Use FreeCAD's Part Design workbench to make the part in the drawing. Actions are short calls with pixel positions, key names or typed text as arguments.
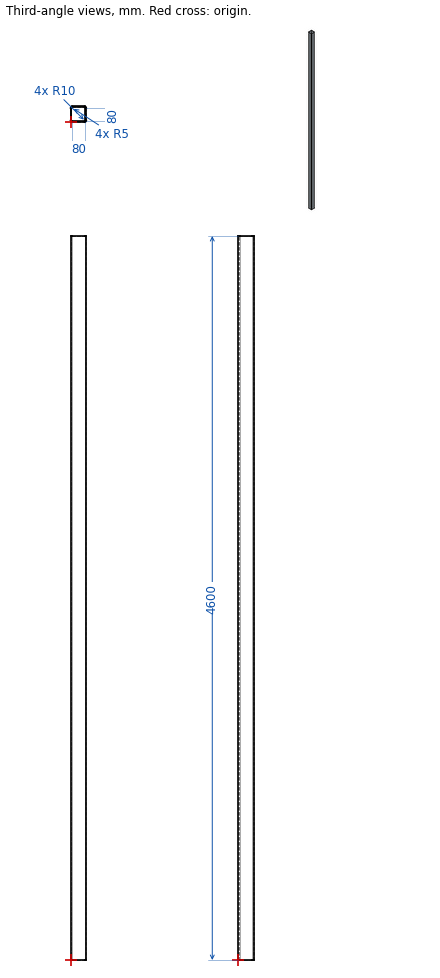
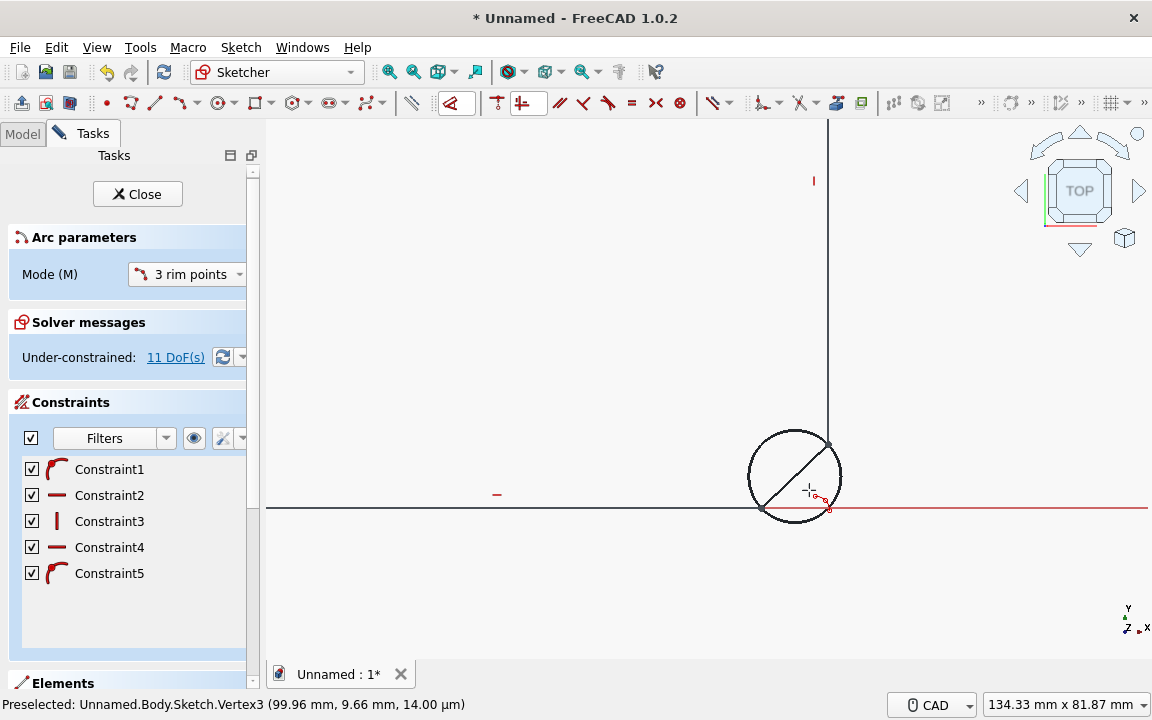
click(809, 489)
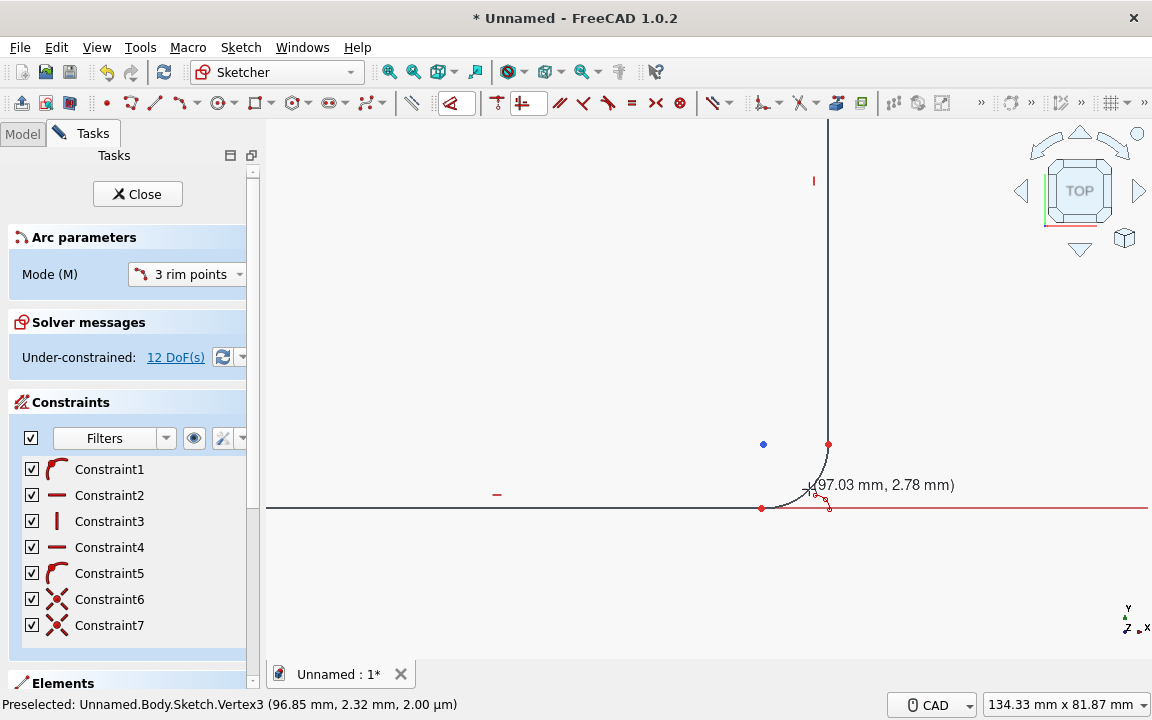
scroll(813, 631, down, 3)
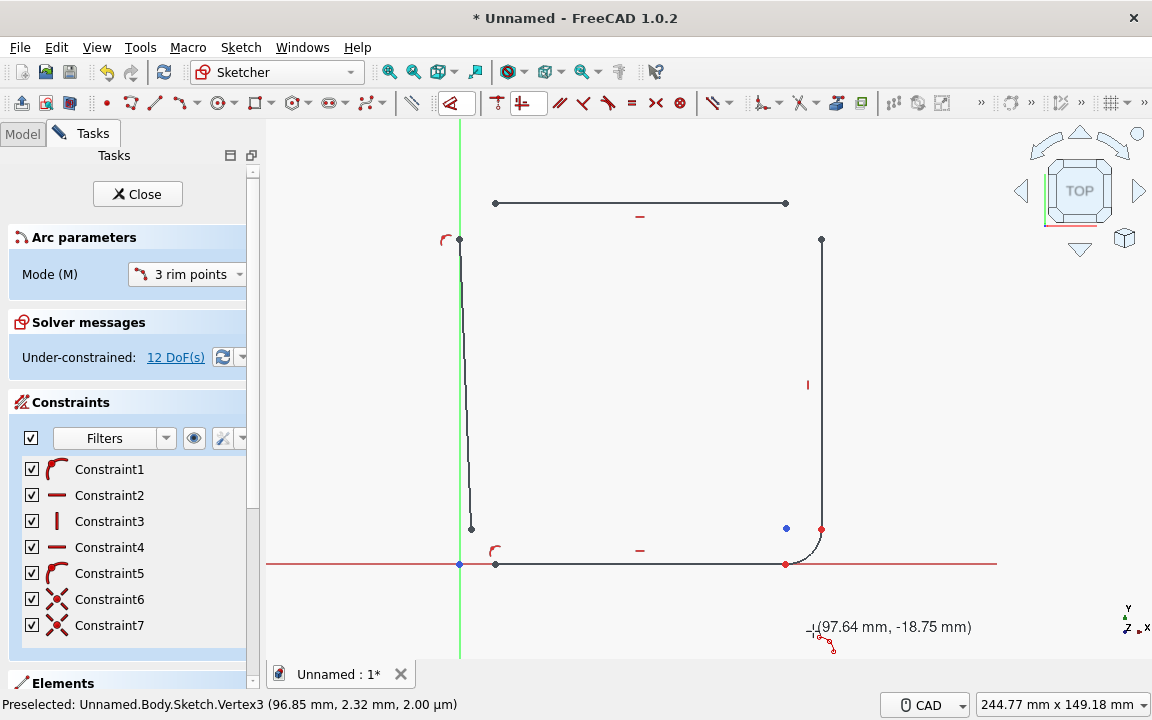
click(822, 240)
click(785, 203)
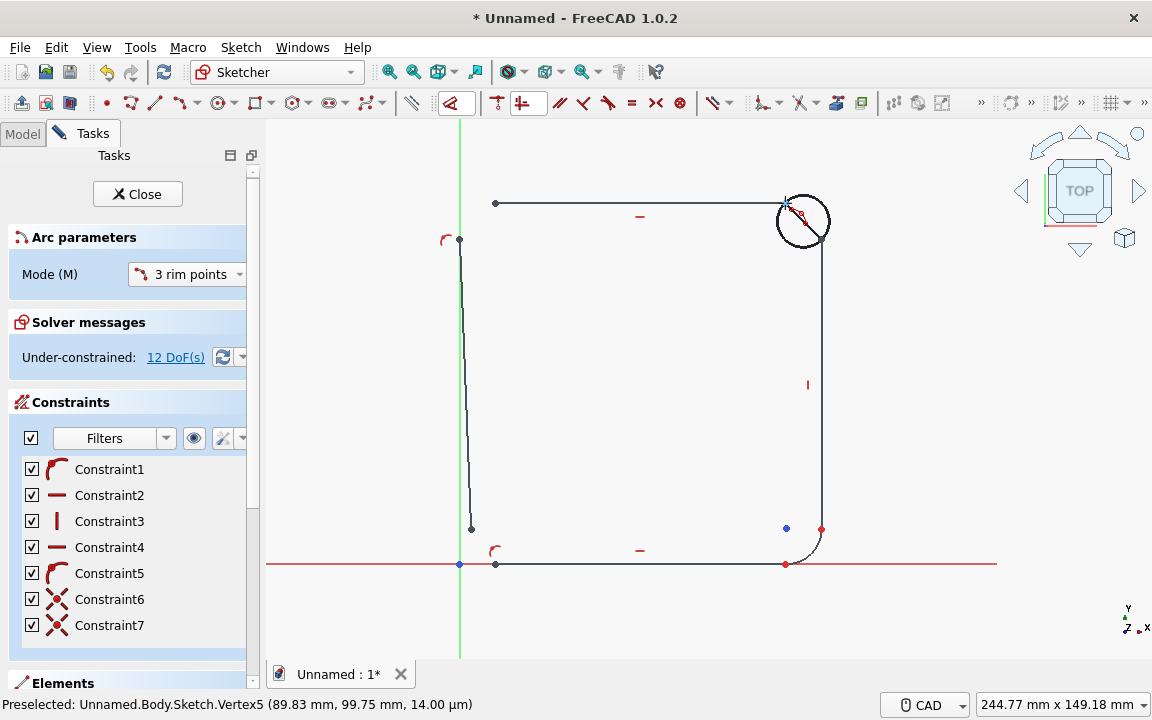
scroll(811, 213, up, 3)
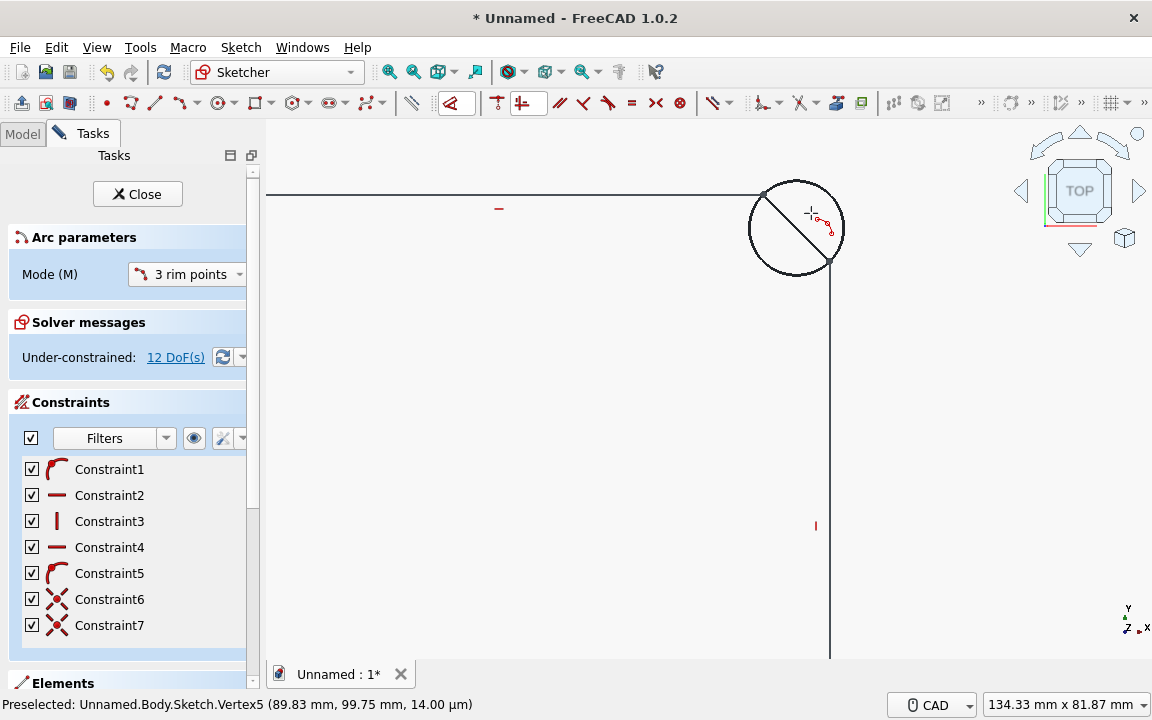
click(811, 212)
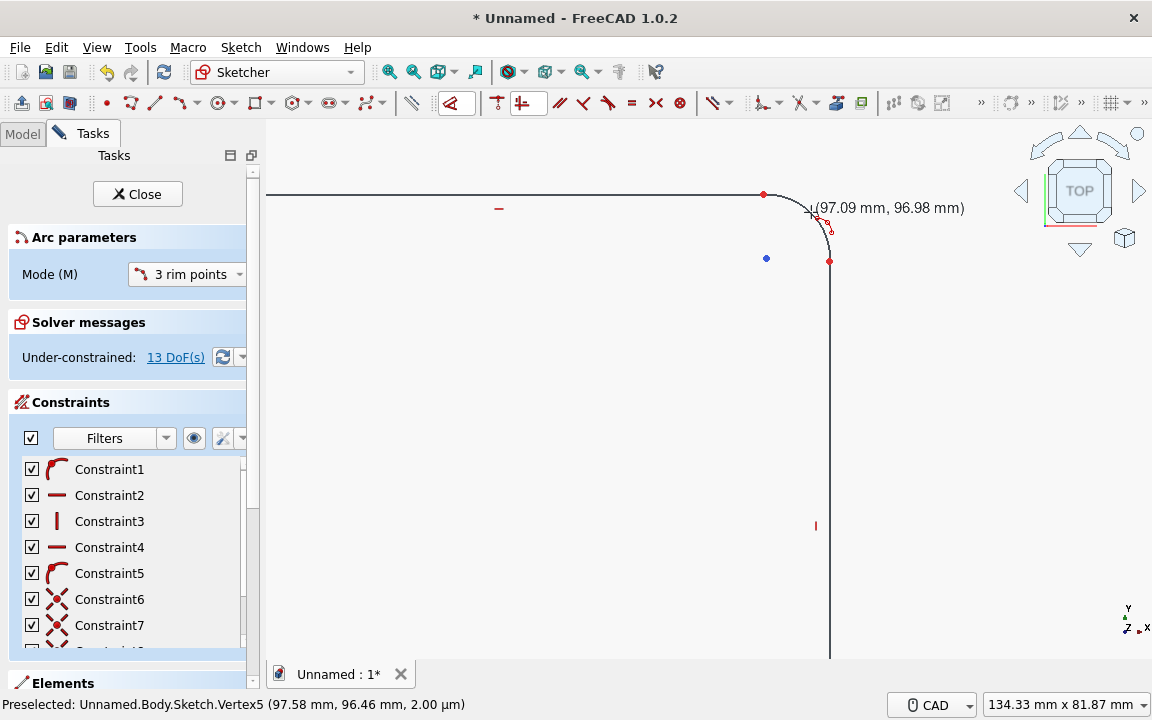
scroll(811, 226, down, 3)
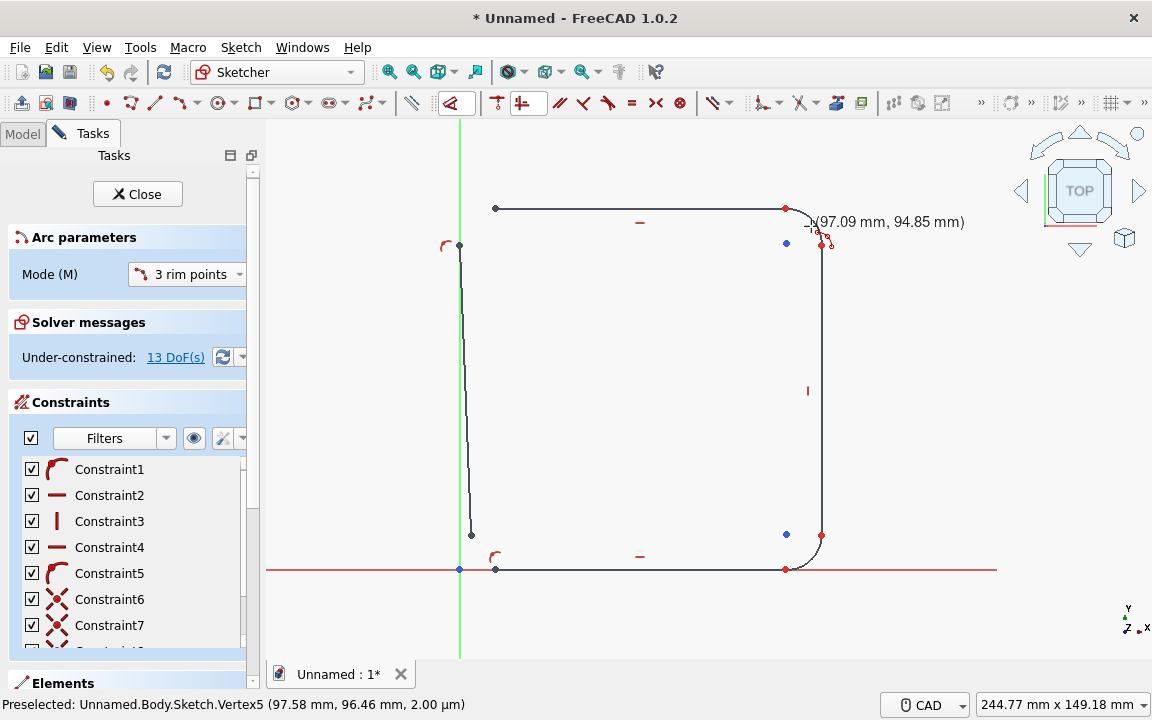
click(496, 209)
click(460, 246)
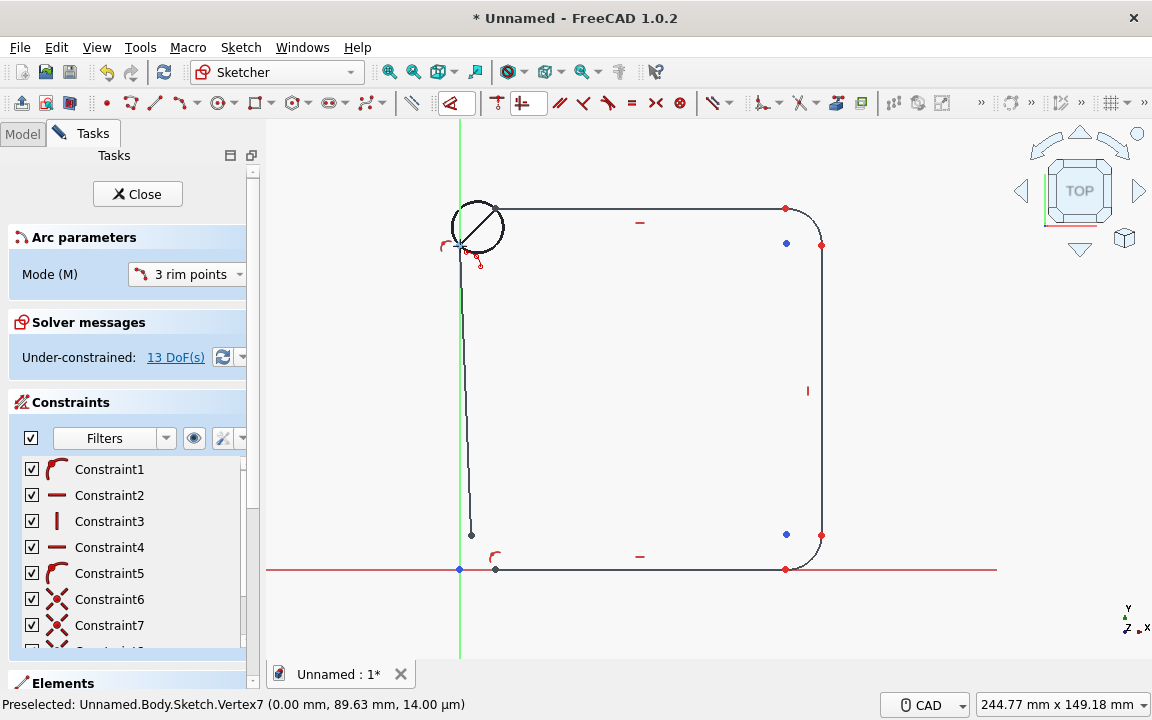
scroll(470, 219, up, 3)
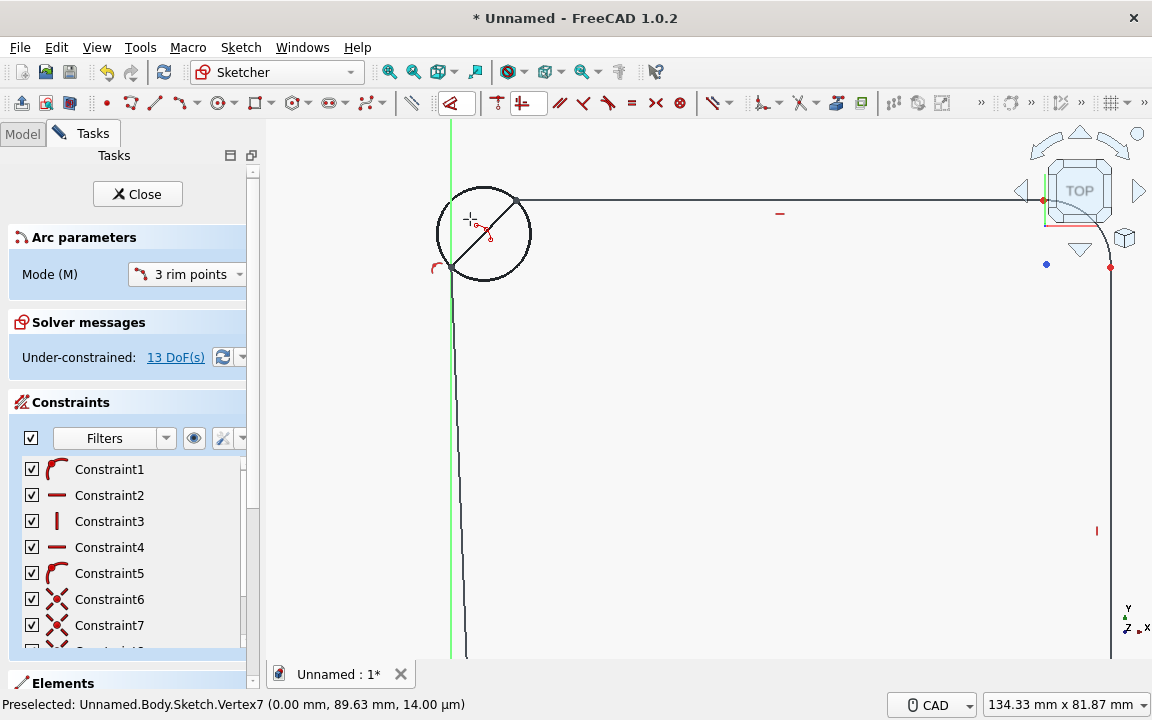
click(471, 218)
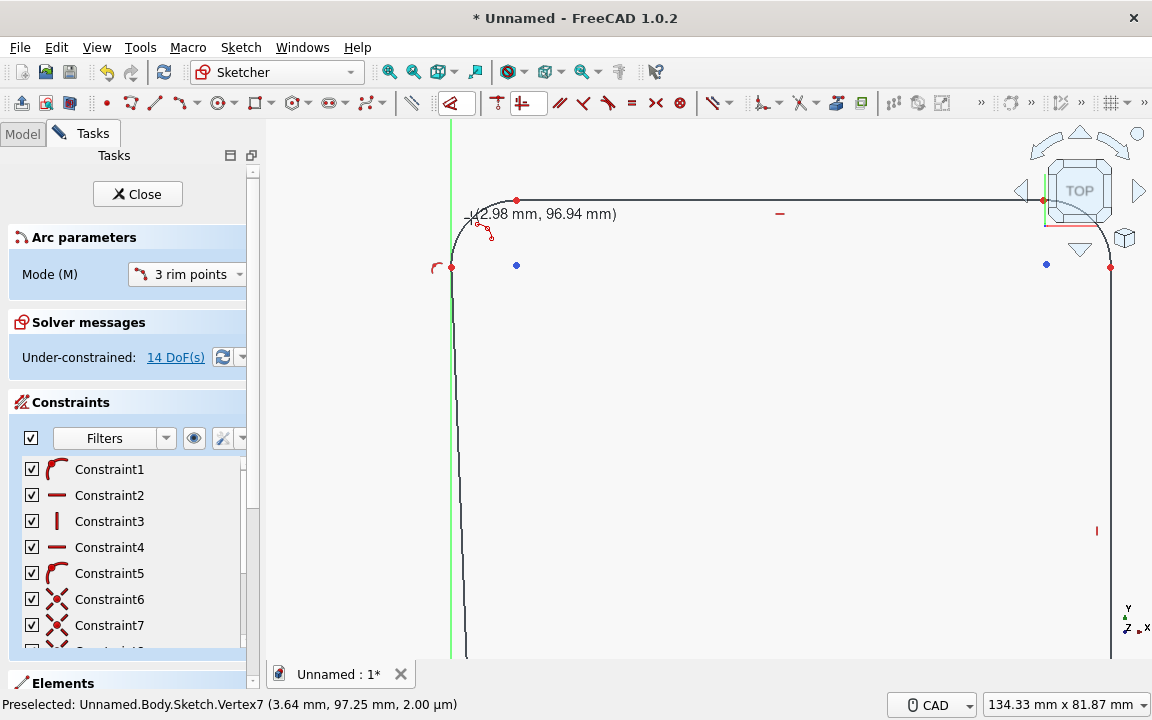
scroll(469, 219, down, 3)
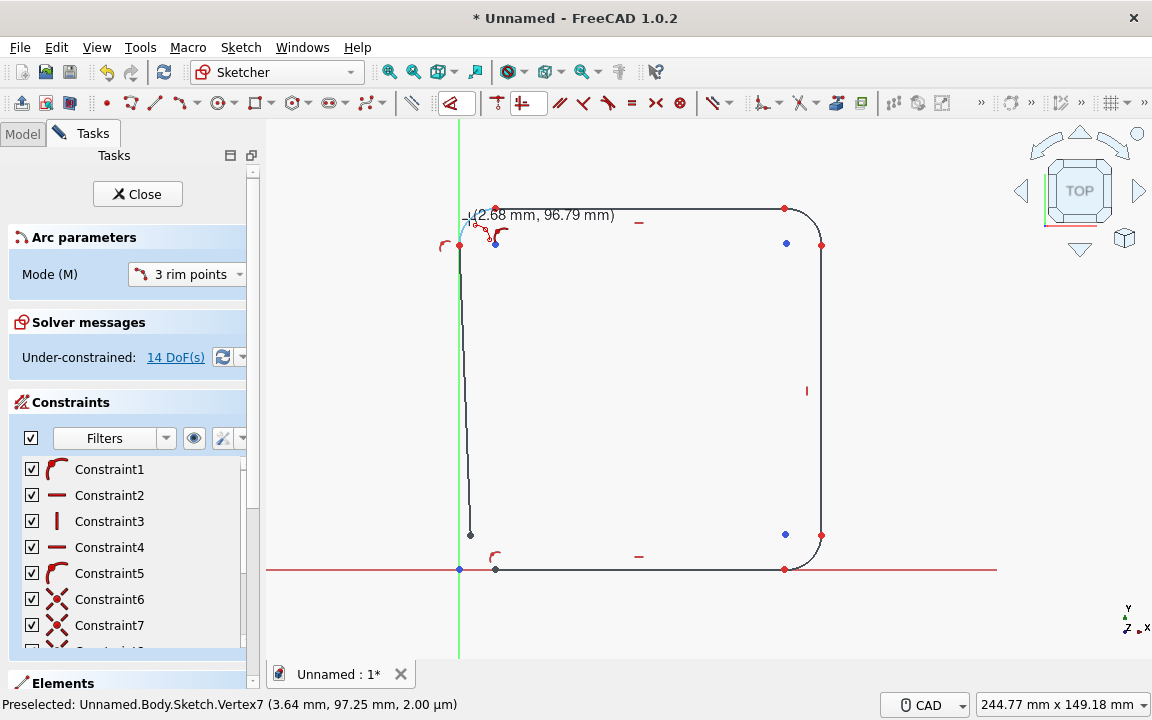
click(471, 535)
click(495, 570)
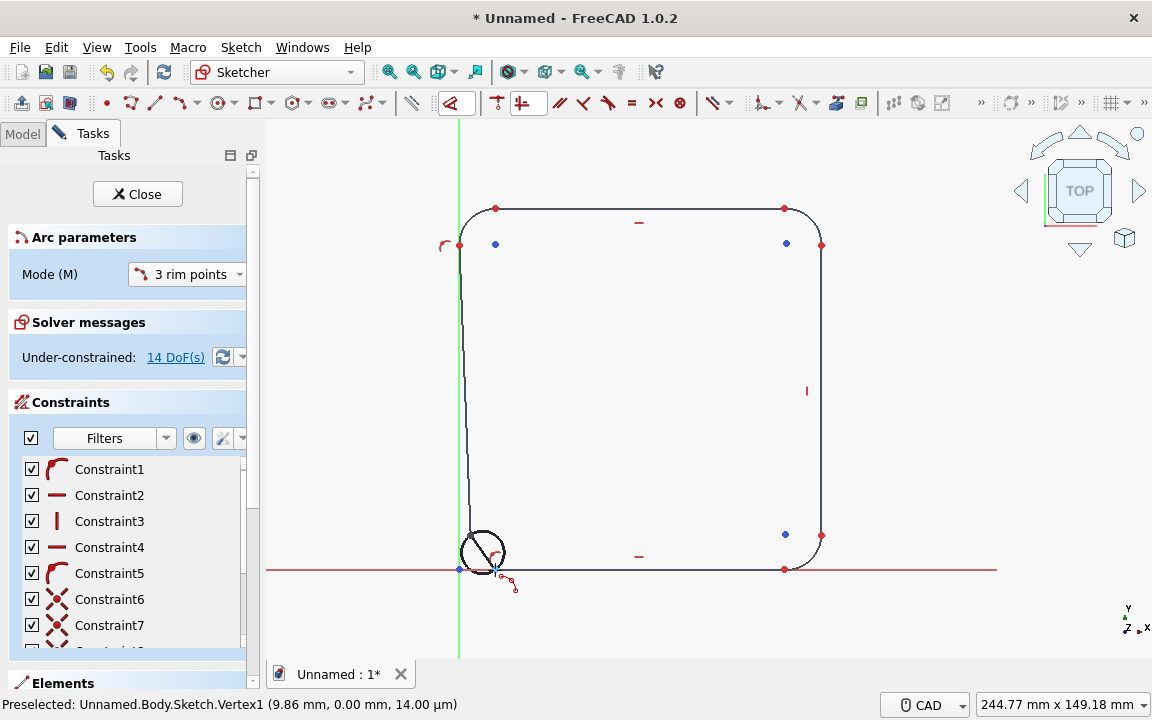
scroll(470, 559, up, 3)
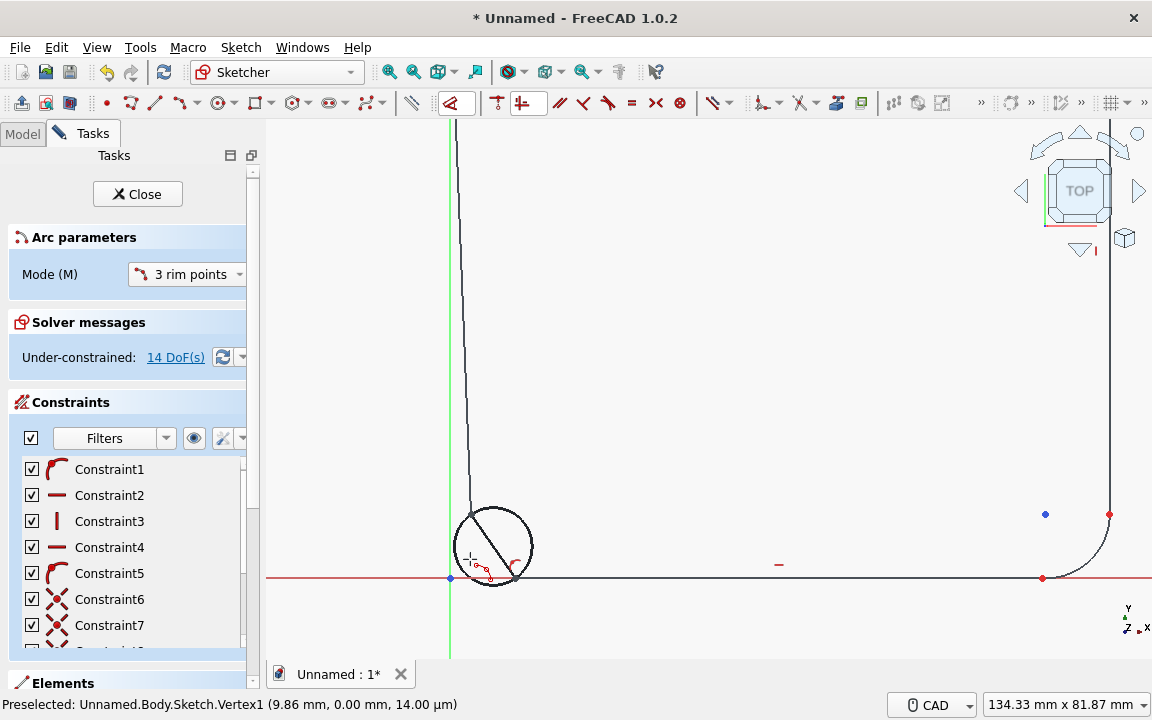
click(470, 559)